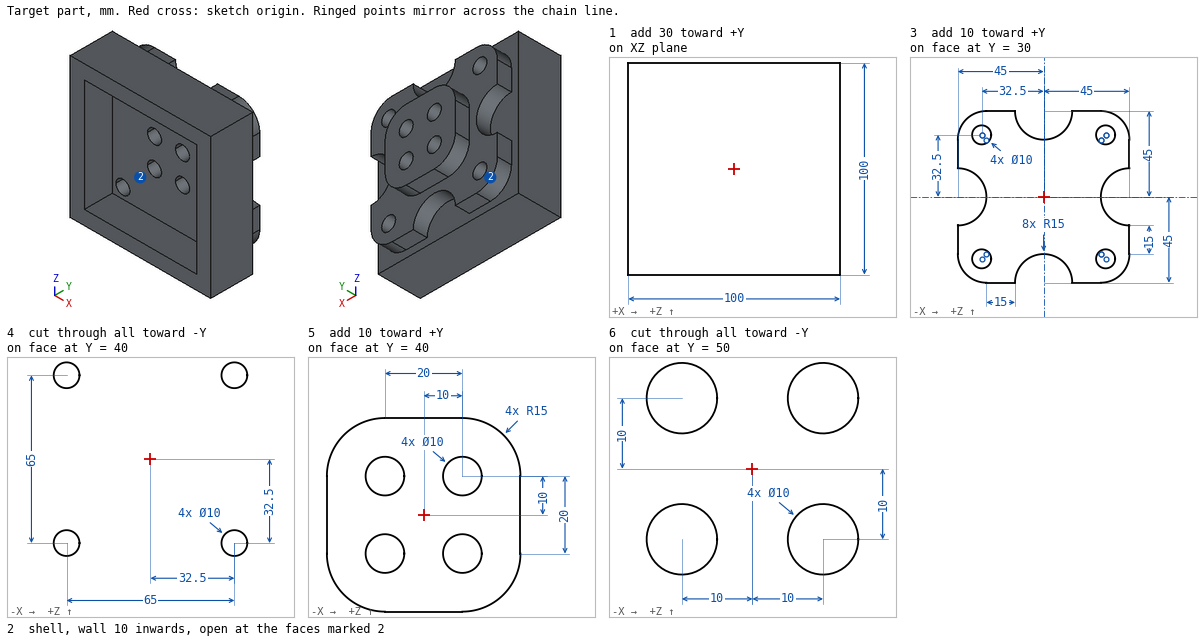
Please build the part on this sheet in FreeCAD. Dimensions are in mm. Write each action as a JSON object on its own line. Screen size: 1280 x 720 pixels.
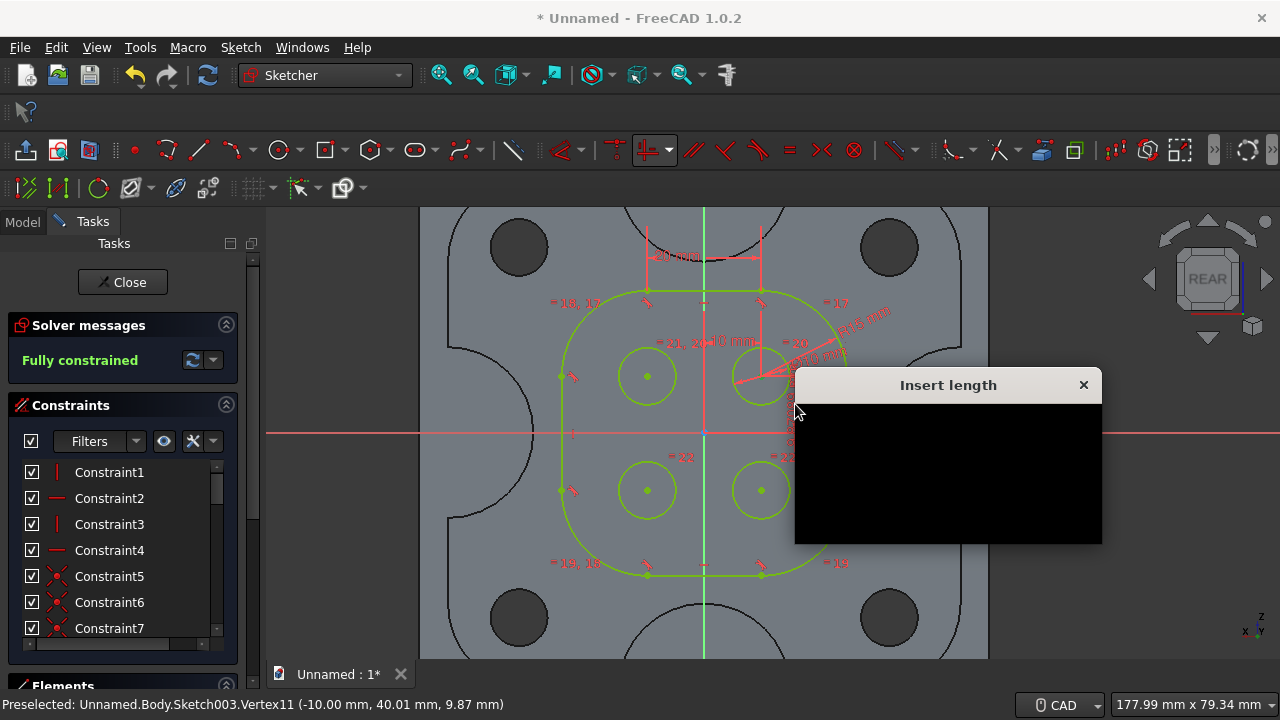
{"action": "type", "text": "10"}
{"action": "key", "text": "Return"}
{"action": "key", "text": "Escape"}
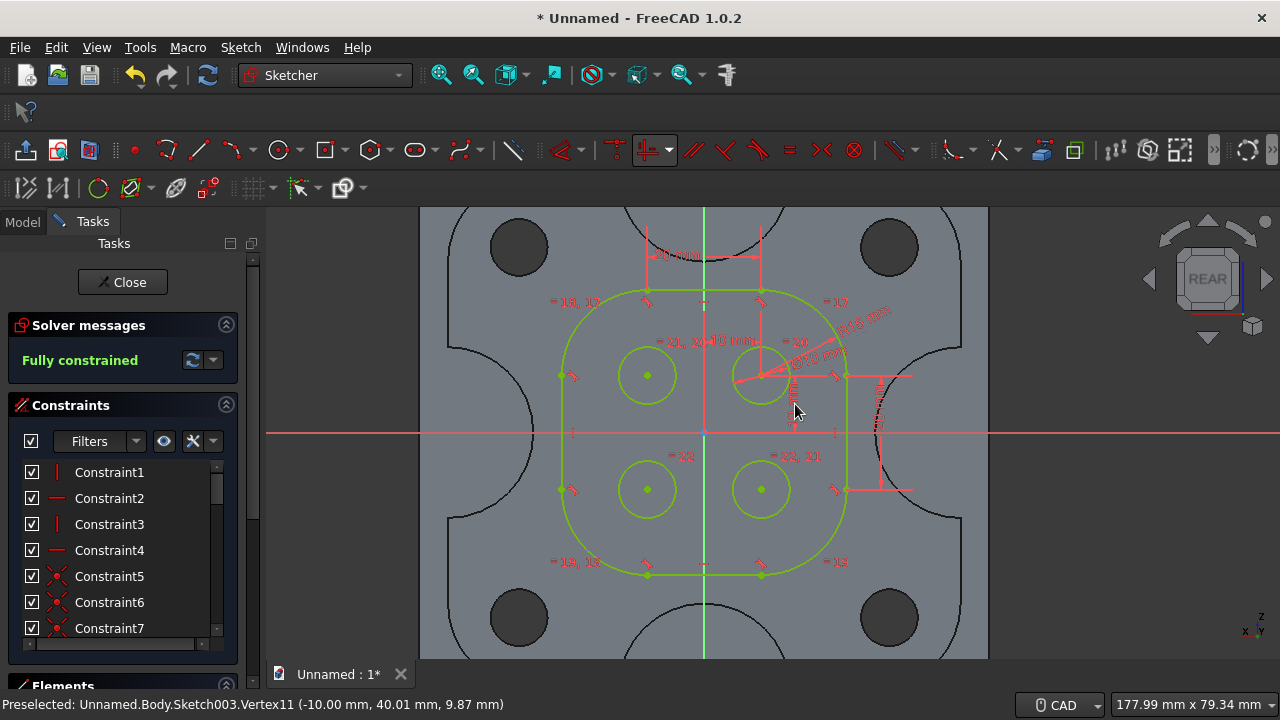
{"action": "left_click", "coordinate": [123, 282]}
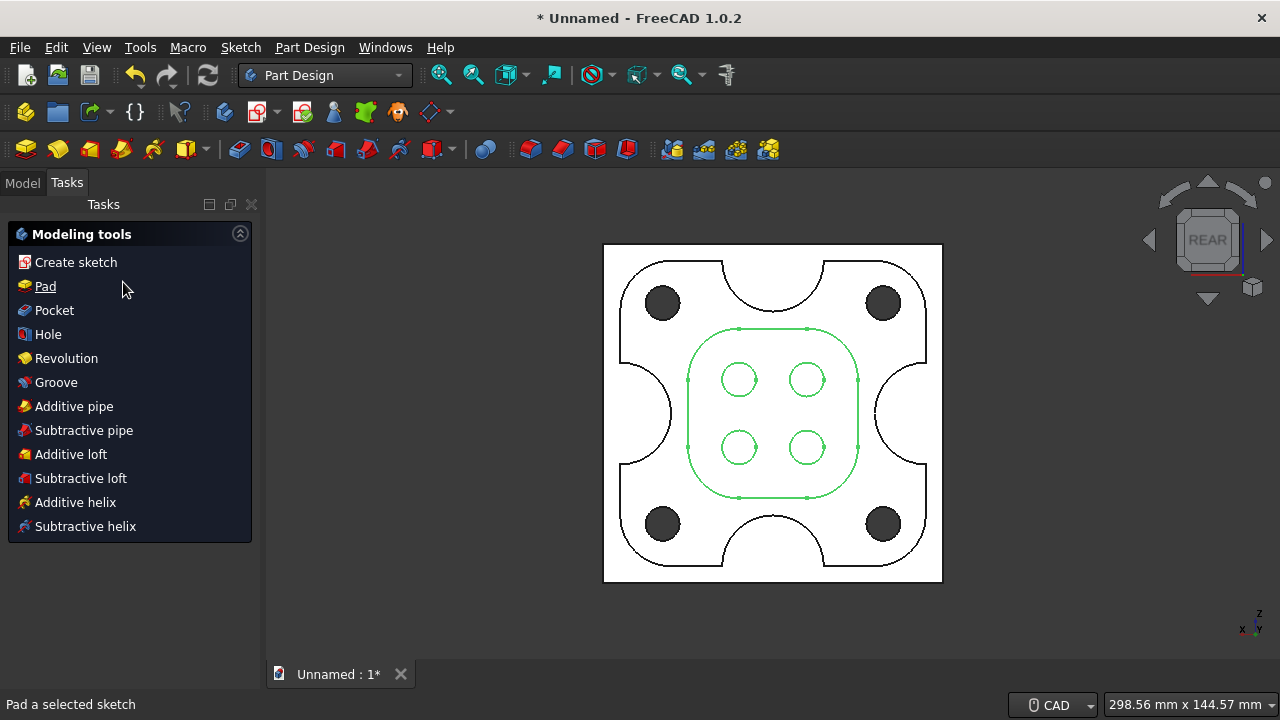
{"action": "left_click", "coordinate": [26, 150]}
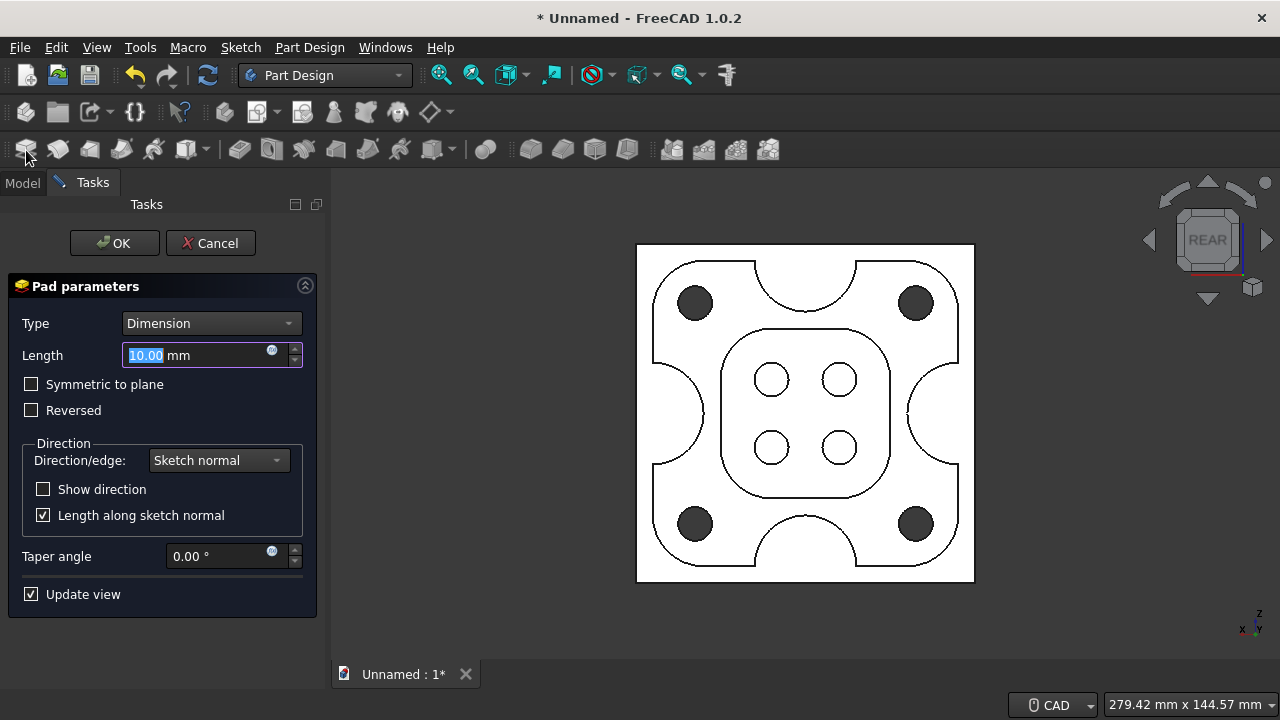
{"action": "type", "text": "10"}
{"action": "key", "text": "Tab"}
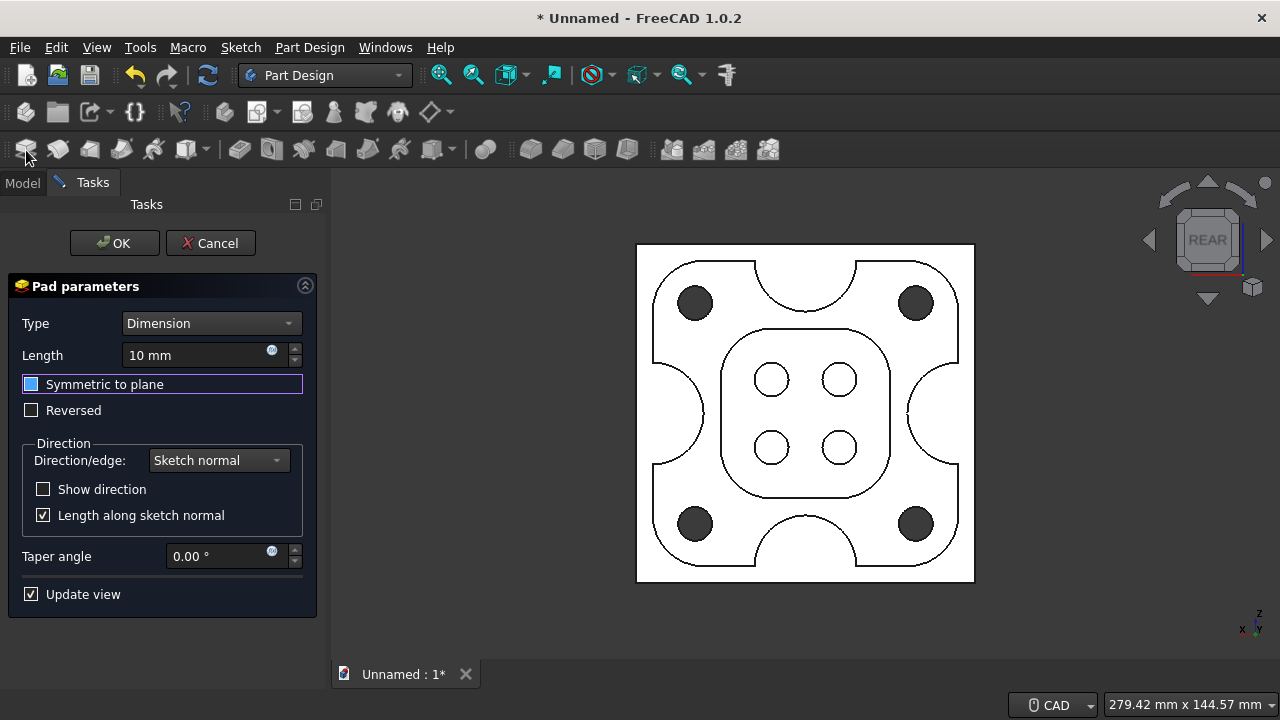
{"action": "left_click", "coordinate": [115, 243]}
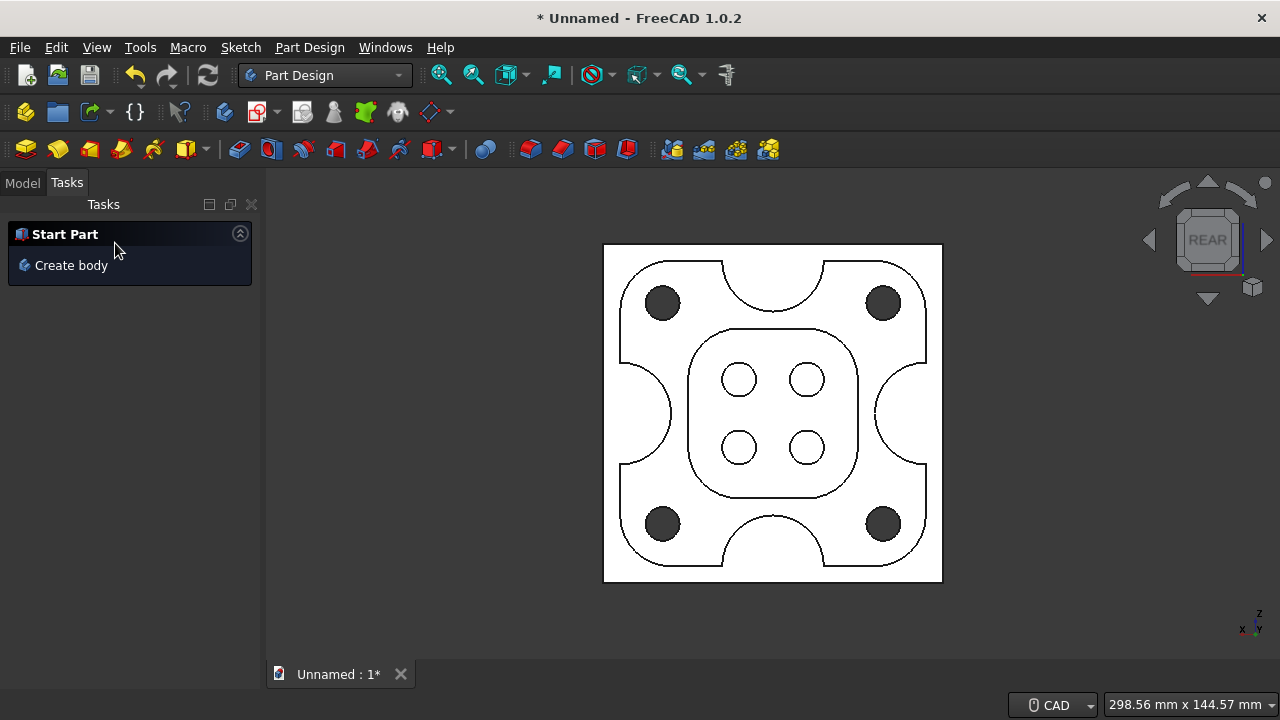
{"action": "left_click", "coordinate": [773, 412]}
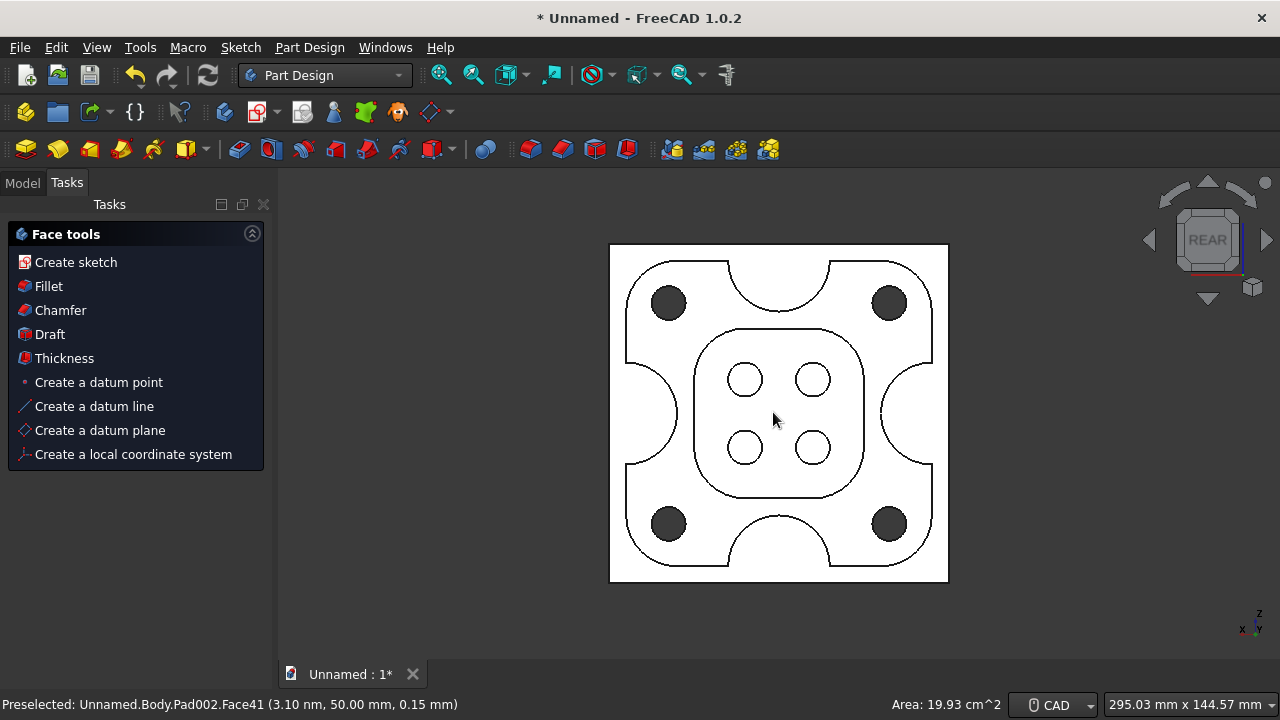
{"action": "left_click", "coordinate": [258, 112]}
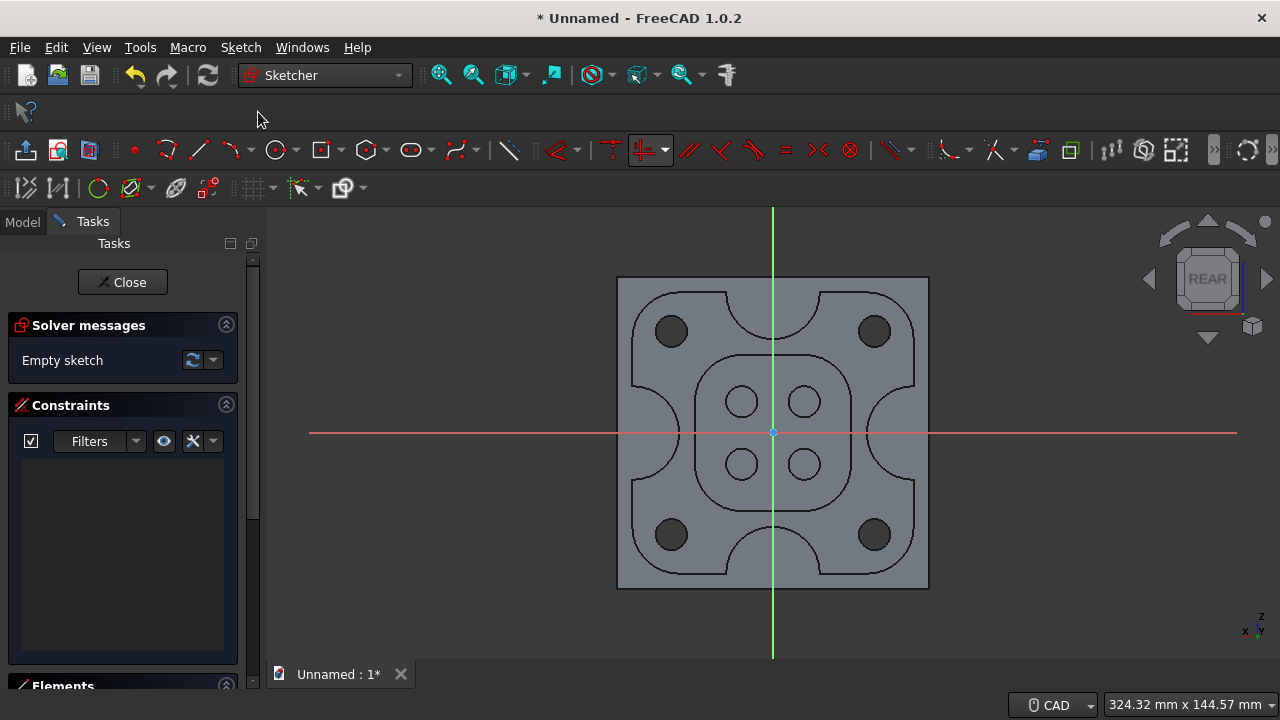
{"action": "scroll", "coordinate": [813, 433], "scroll_direction": "up", "scroll_amount": 5}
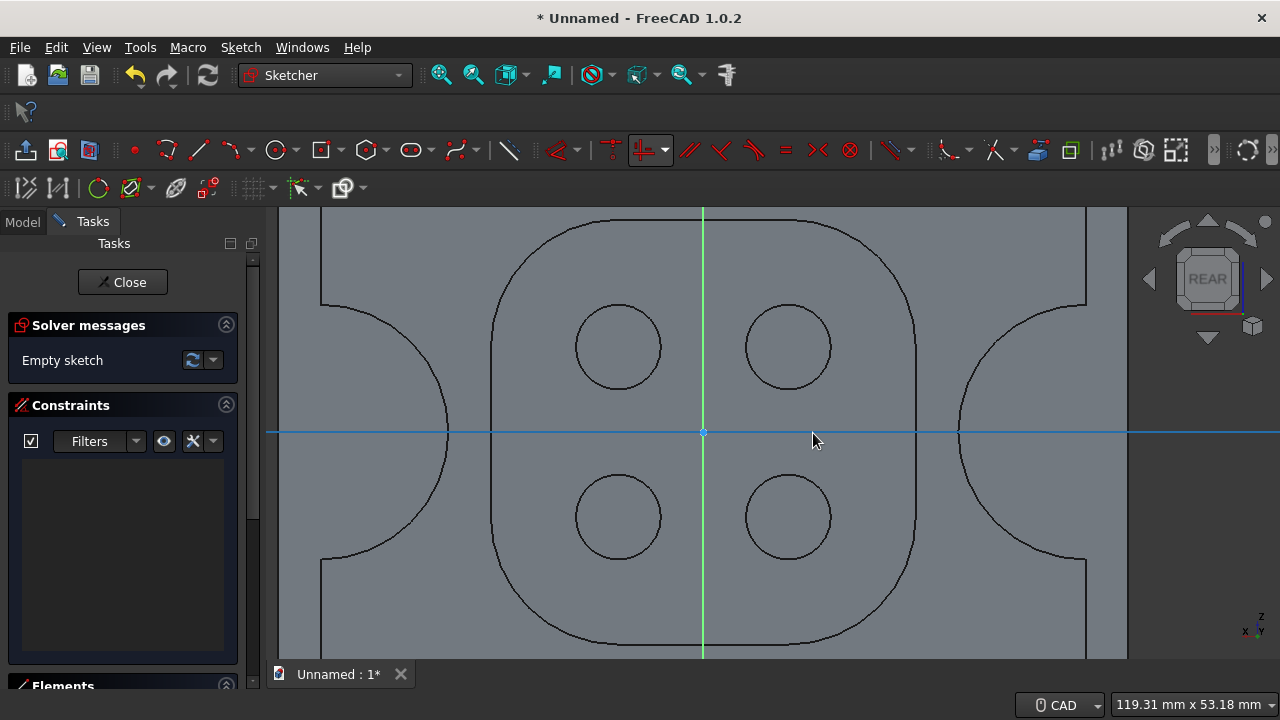
{"action": "left_click", "coordinate": [276, 150]}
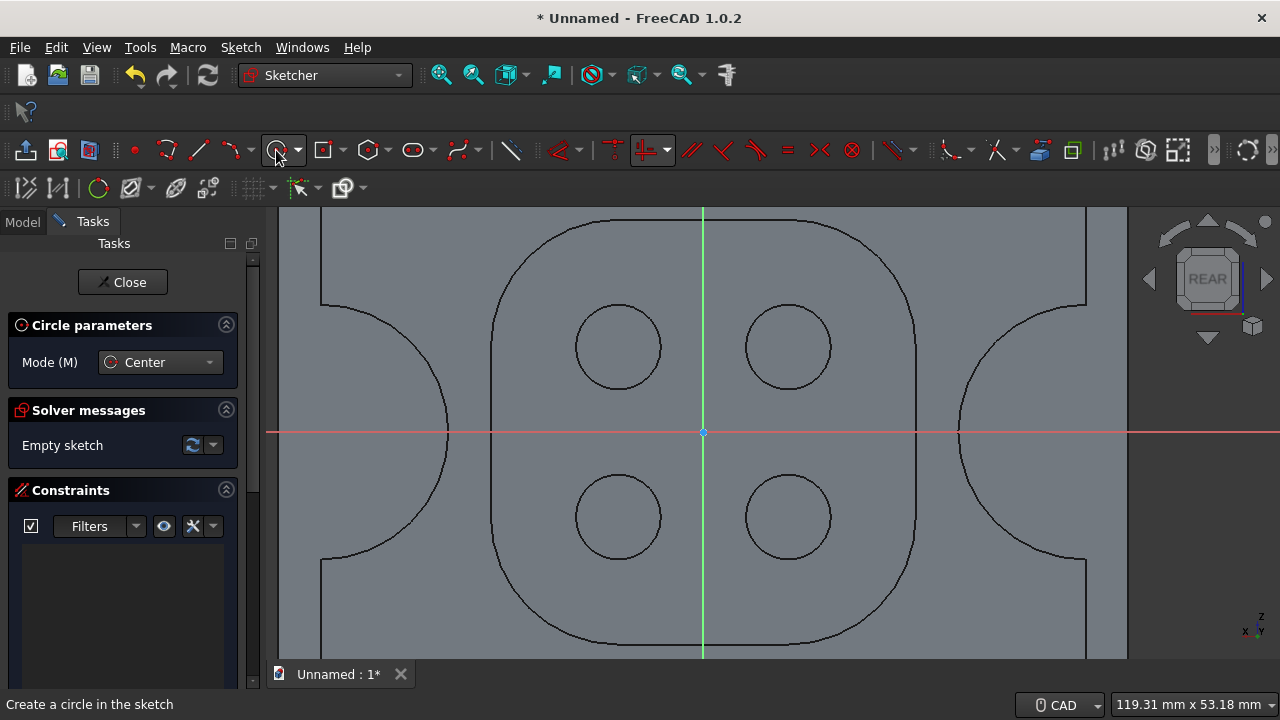
{"action": "left_click", "coordinate": [788, 517]}
{"action": "left_click", "coordinate": [818, 487]}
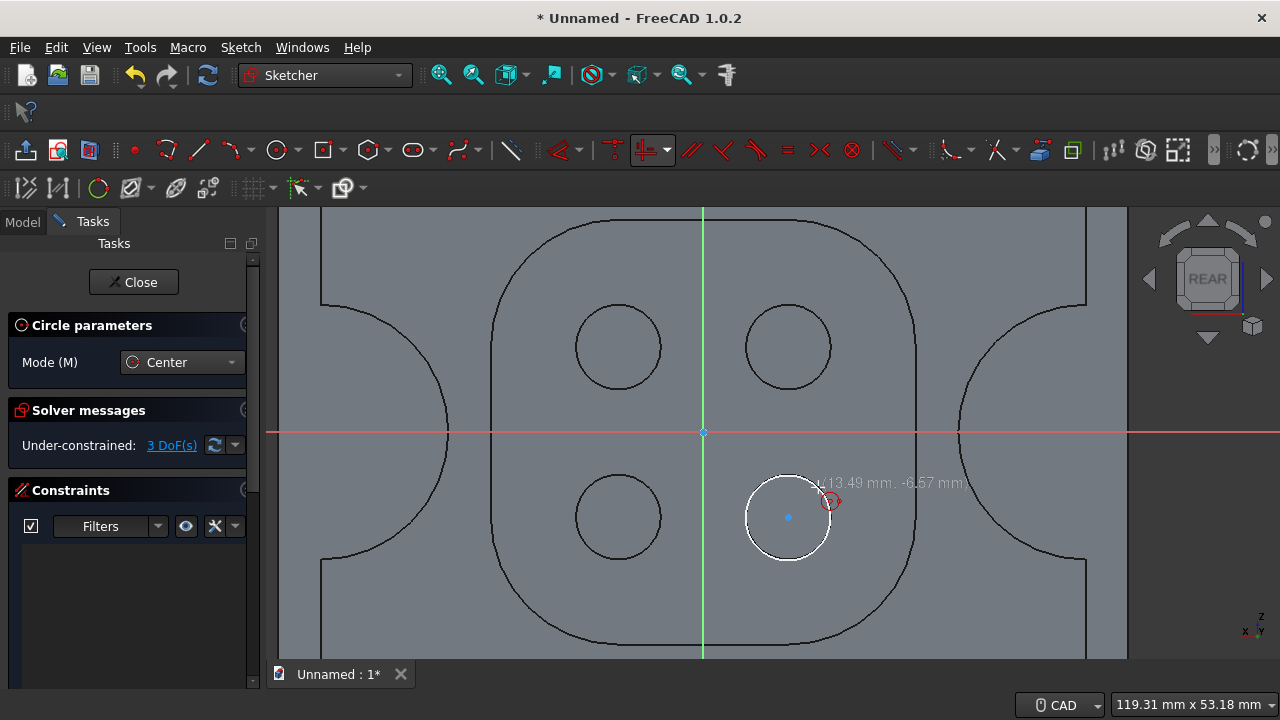
{"action": "left_click", "coordinate": [618, 517]}
{"action": "left_click", "coordinate": [648, 487]}